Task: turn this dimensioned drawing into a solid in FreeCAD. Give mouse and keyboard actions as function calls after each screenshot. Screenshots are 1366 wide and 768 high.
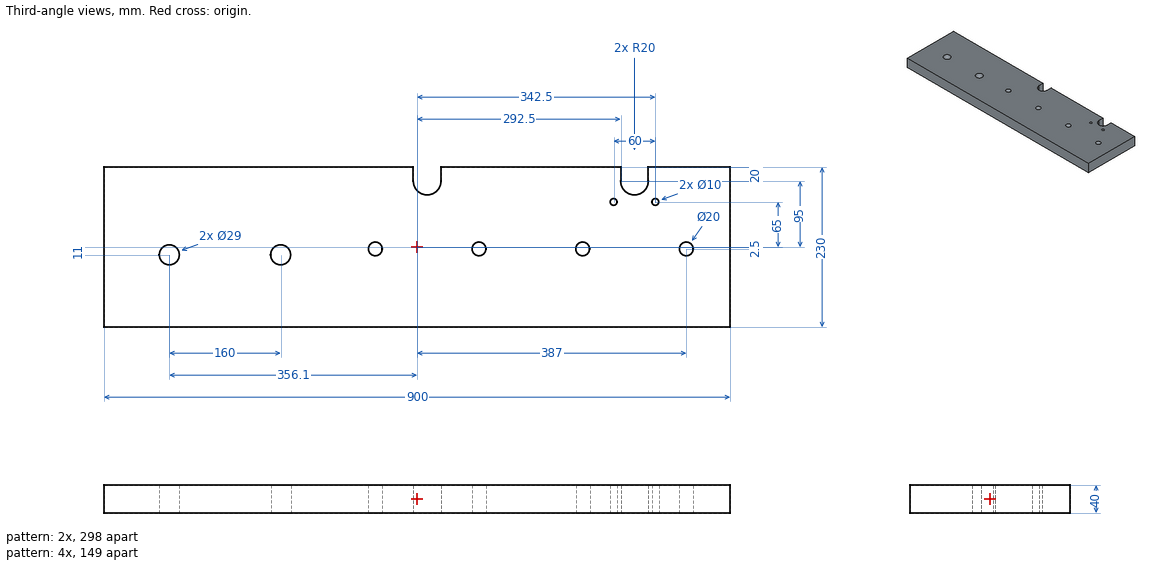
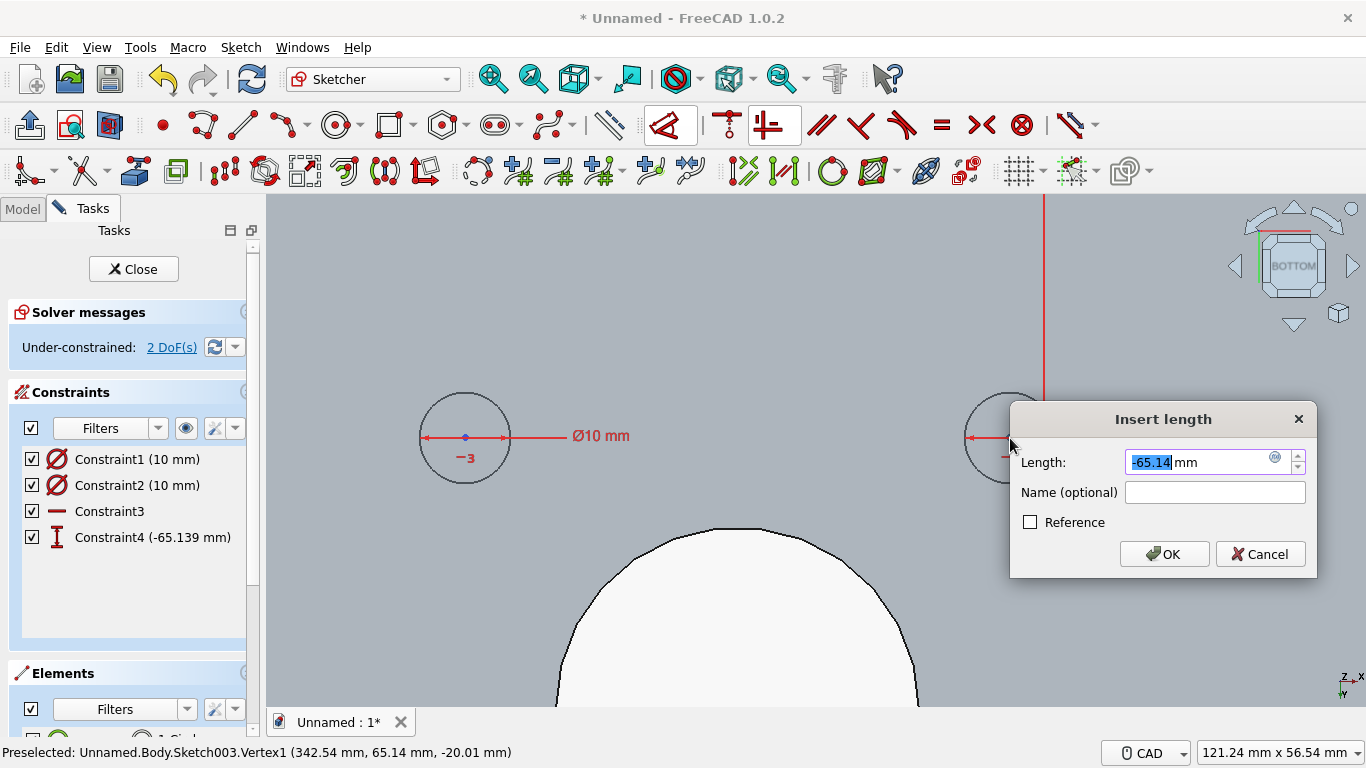
text(-65)
key(Return)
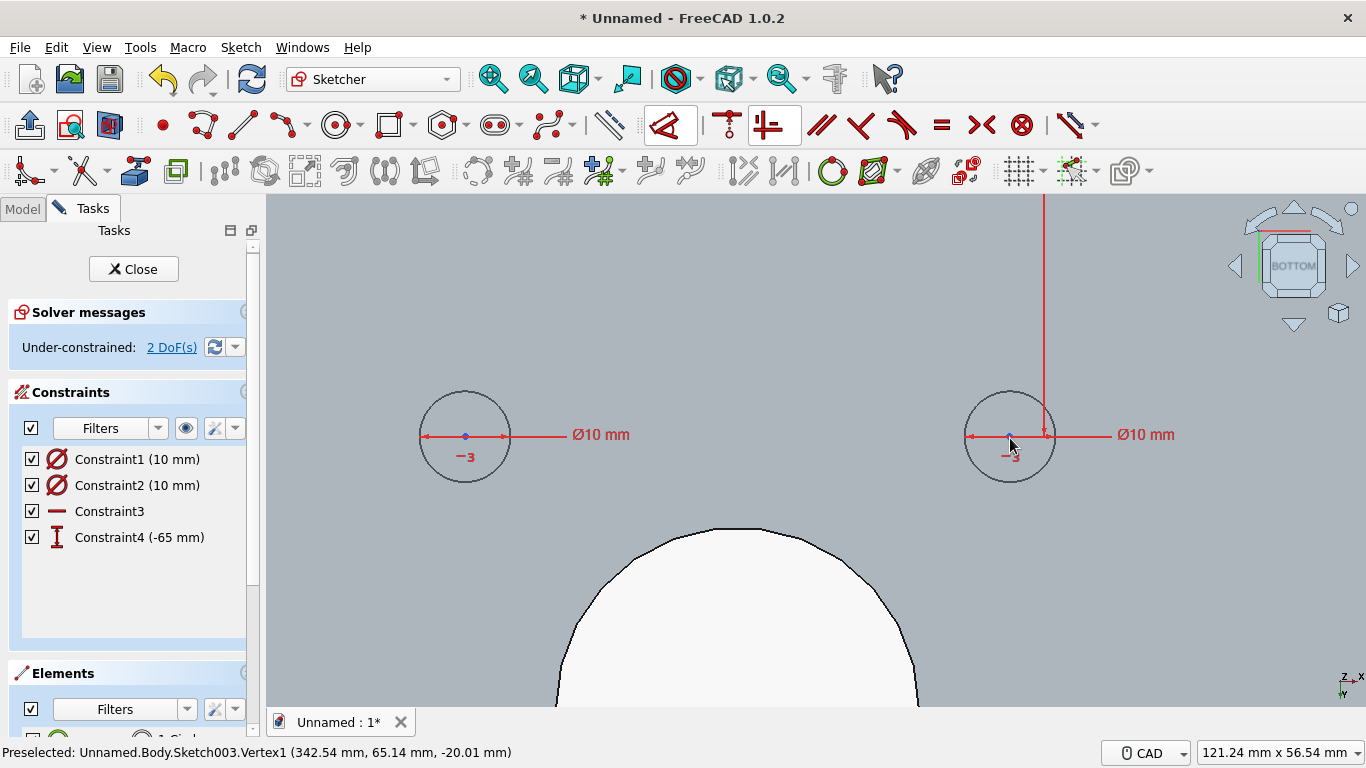
click(1010, 437)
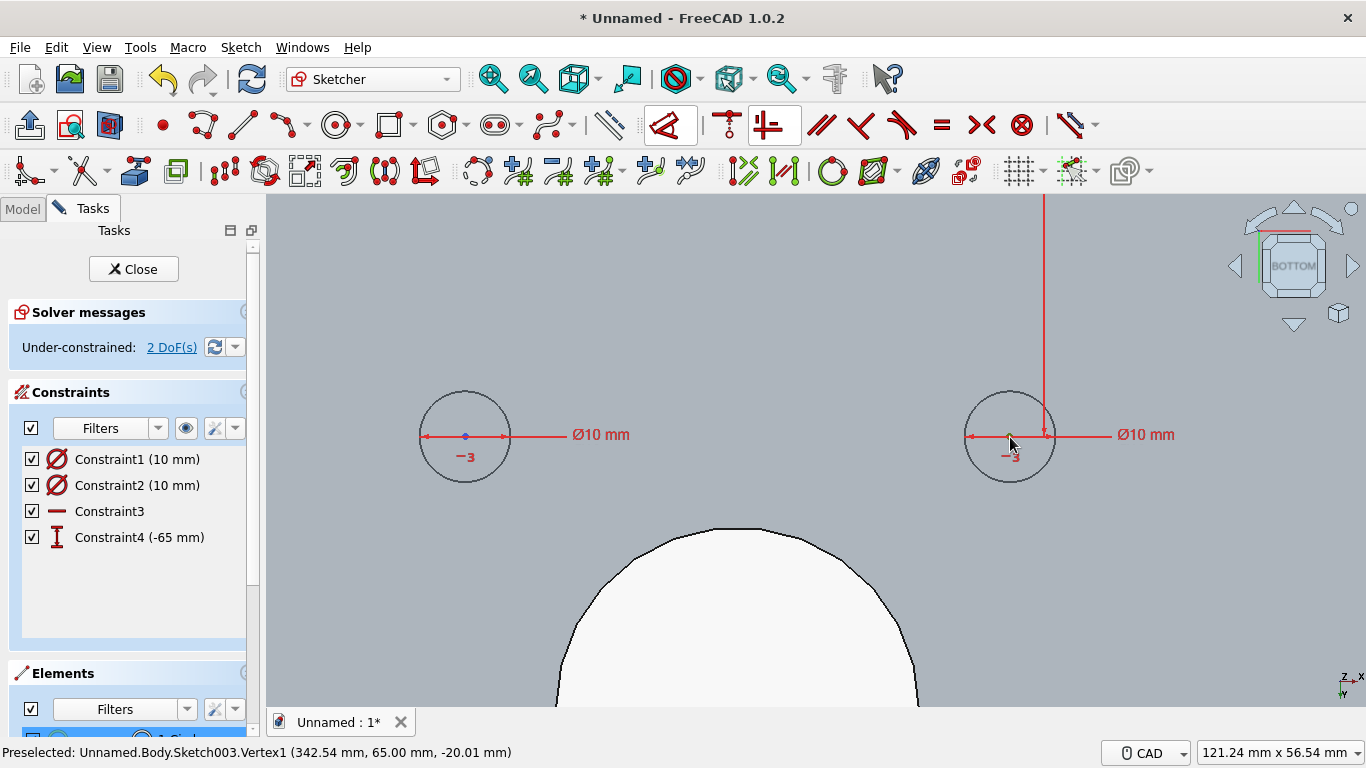
click(465, 437)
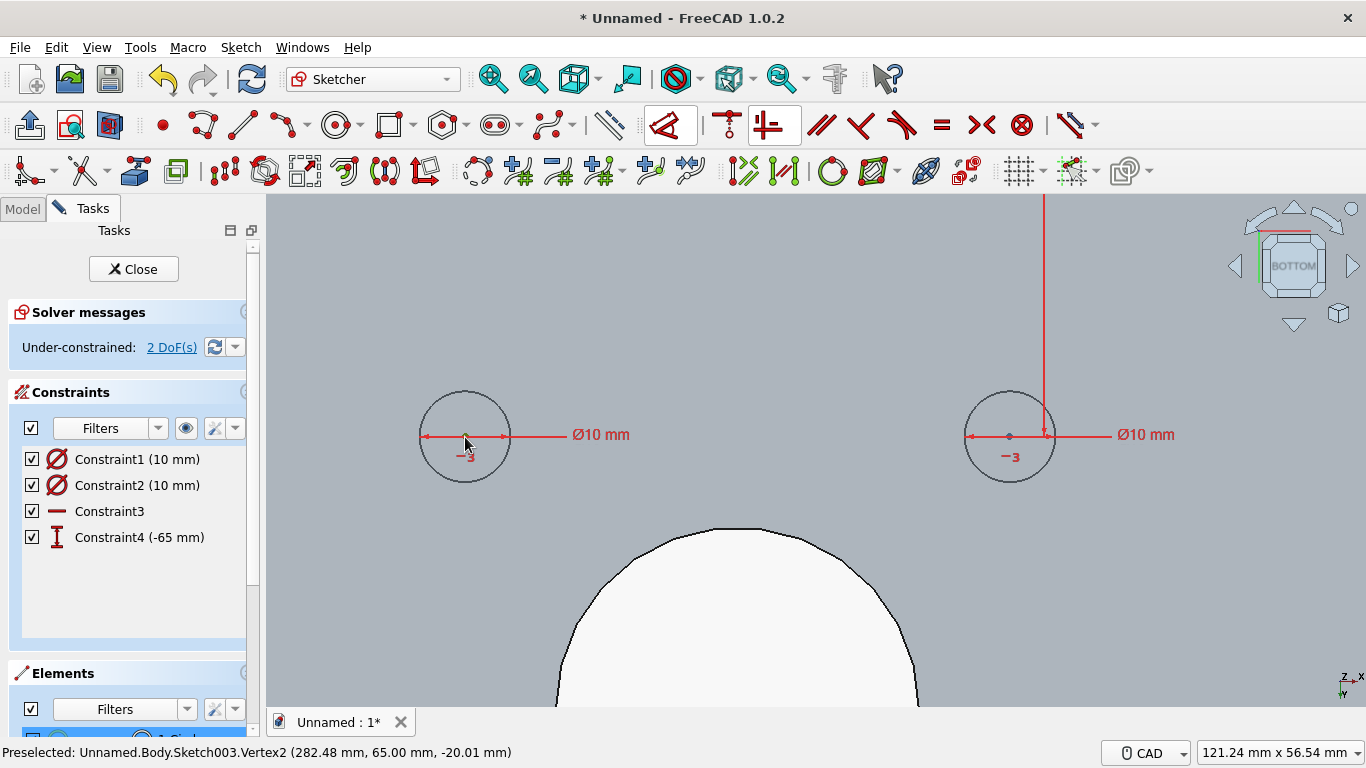
key(l)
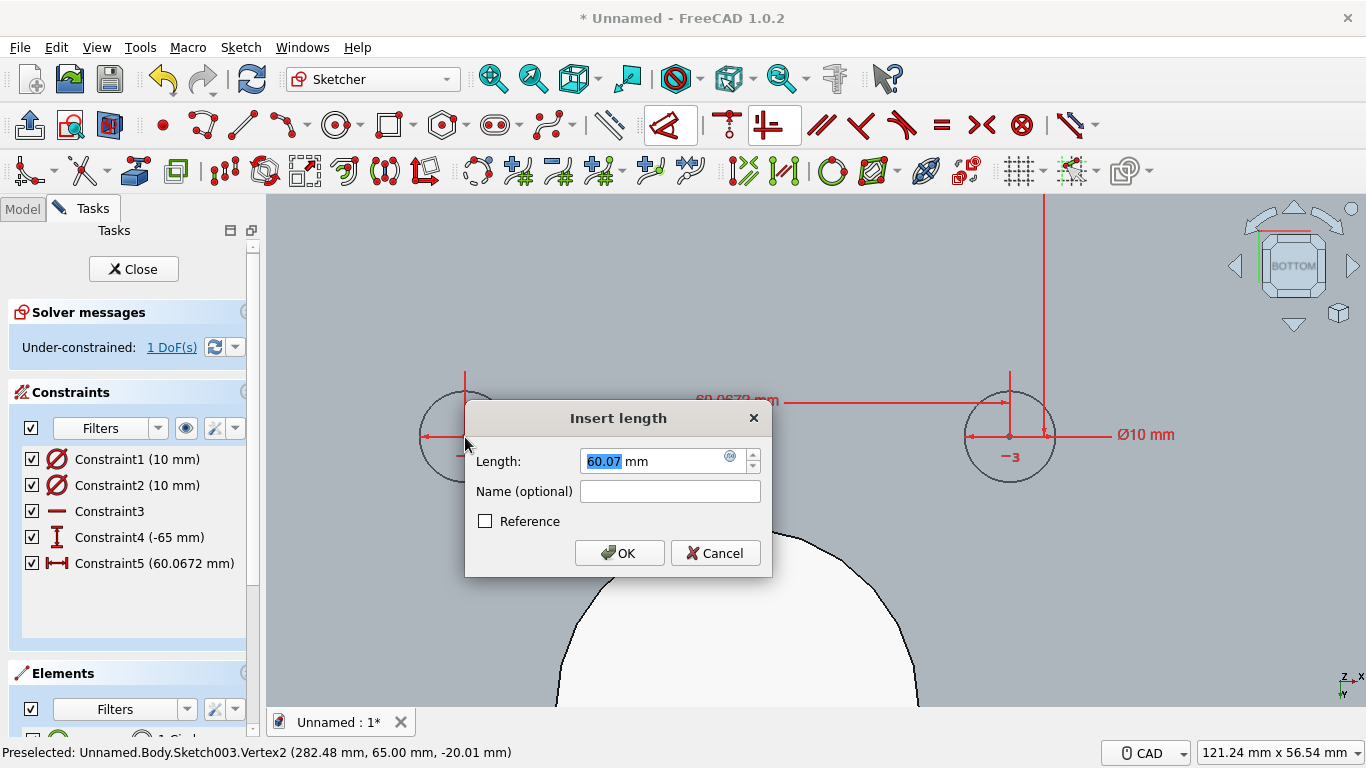
text(60)
key(Return)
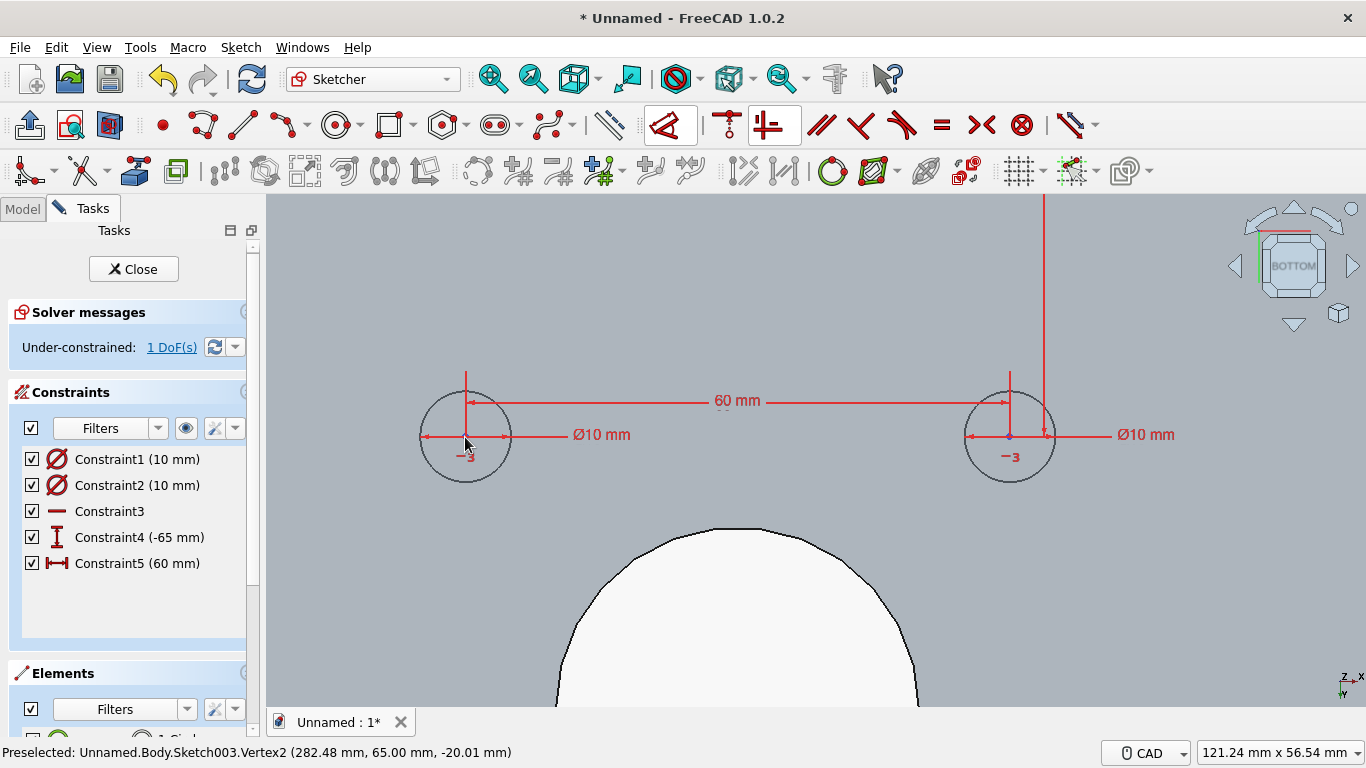
click(1010, 437)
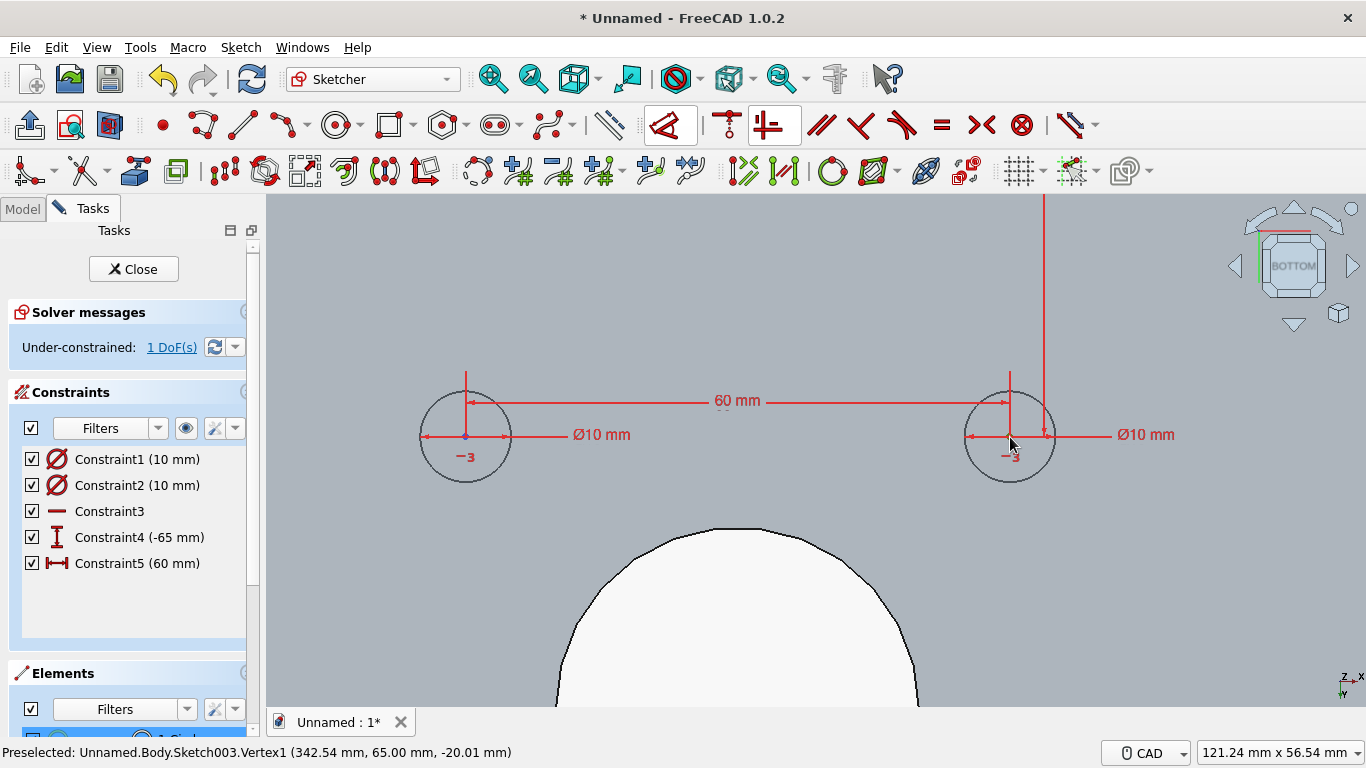
key(l)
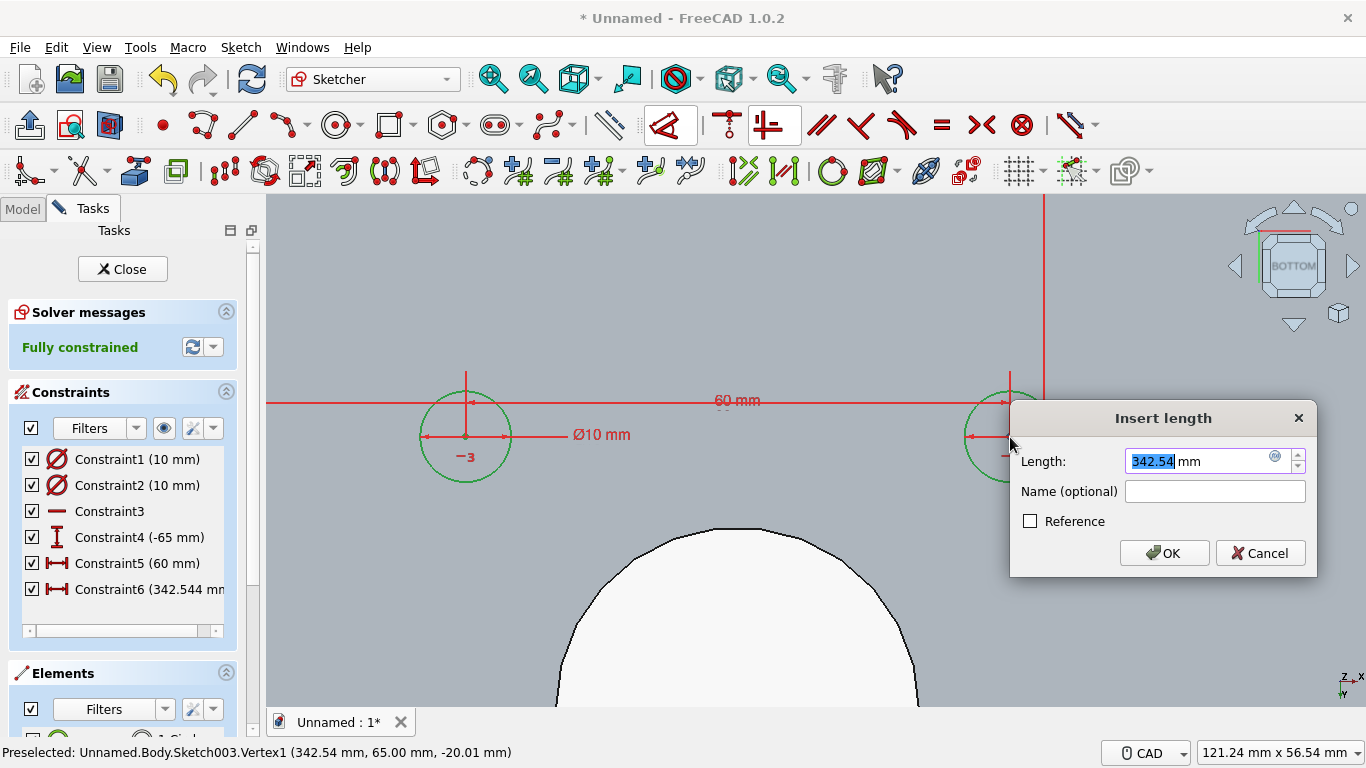
text(342.5)
key(Return)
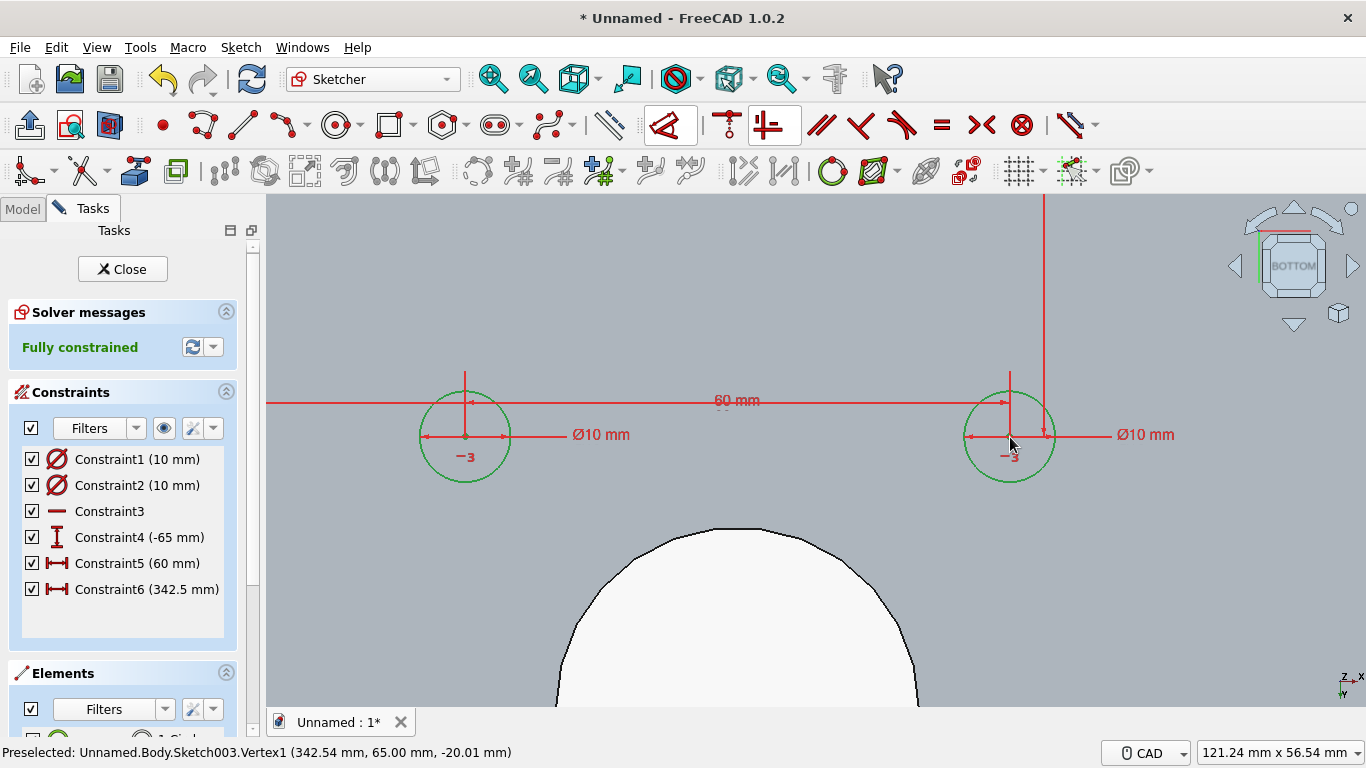
click(123, 269)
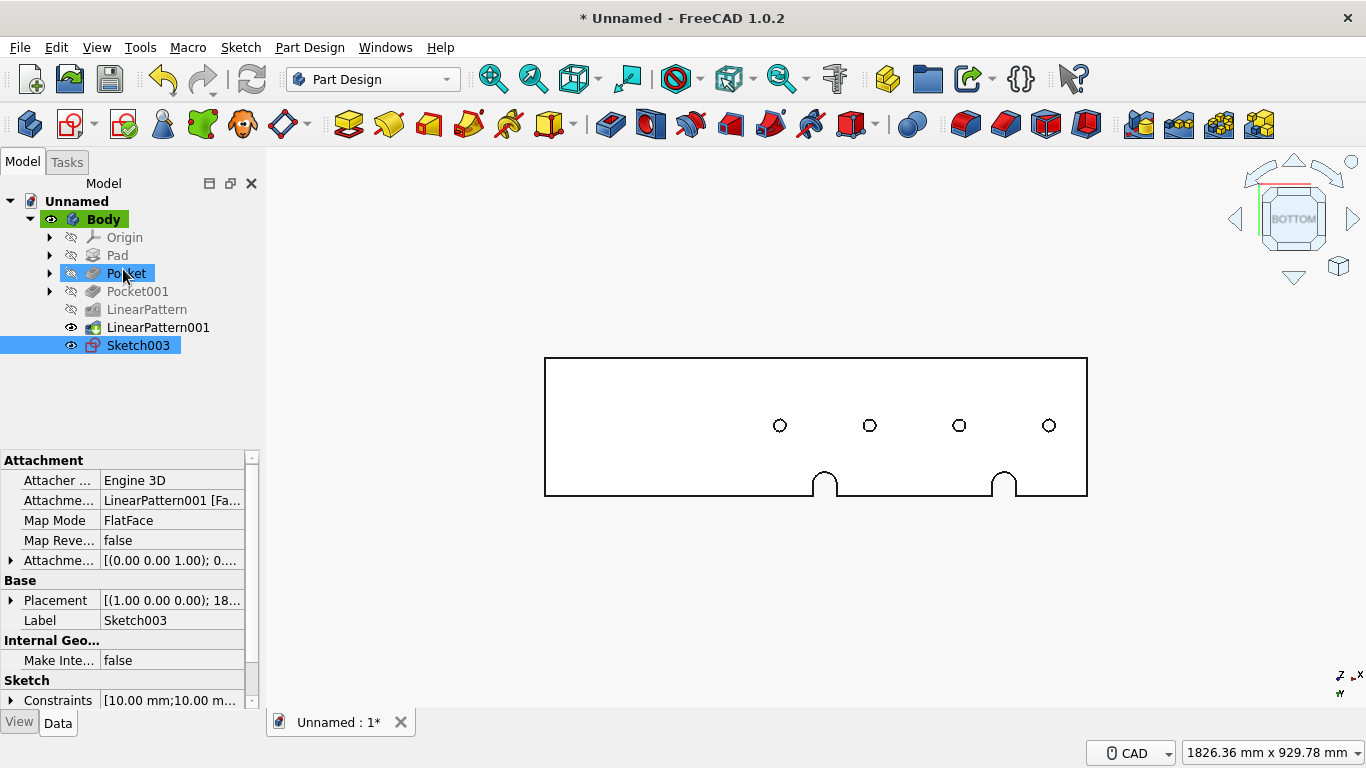
click(612, 124)